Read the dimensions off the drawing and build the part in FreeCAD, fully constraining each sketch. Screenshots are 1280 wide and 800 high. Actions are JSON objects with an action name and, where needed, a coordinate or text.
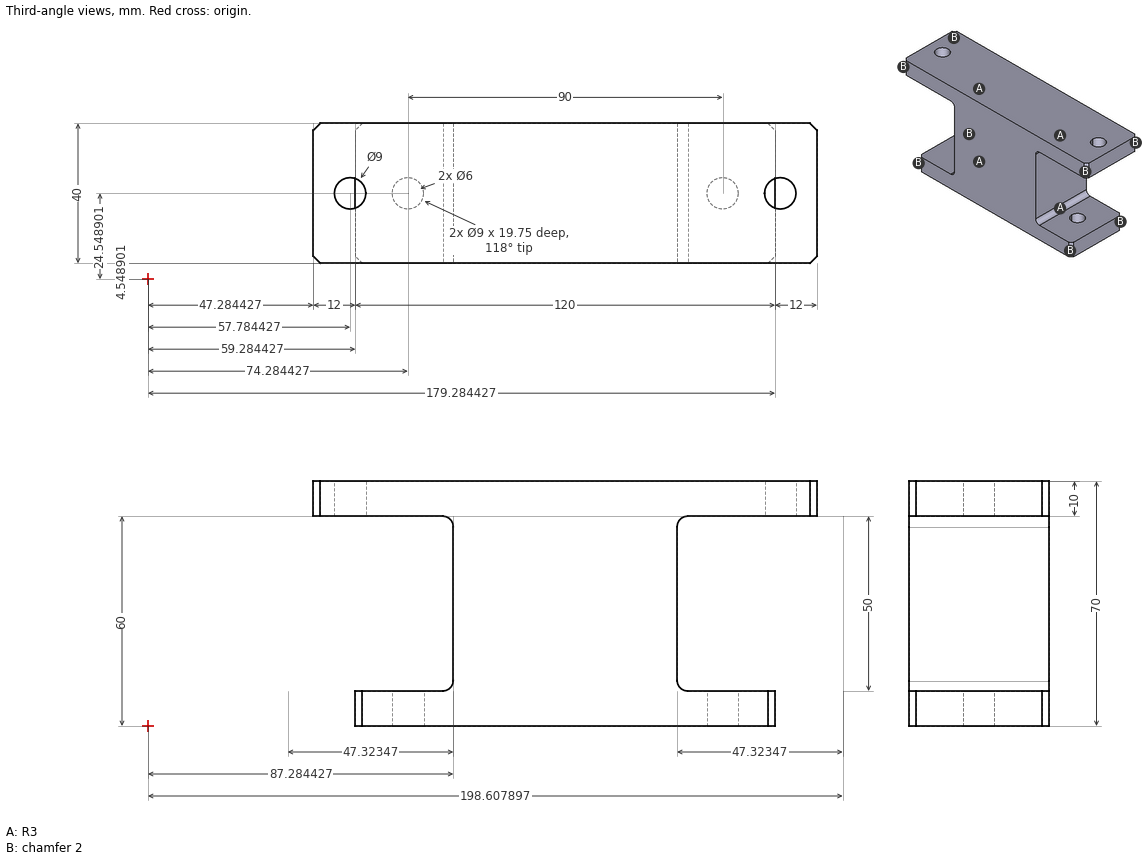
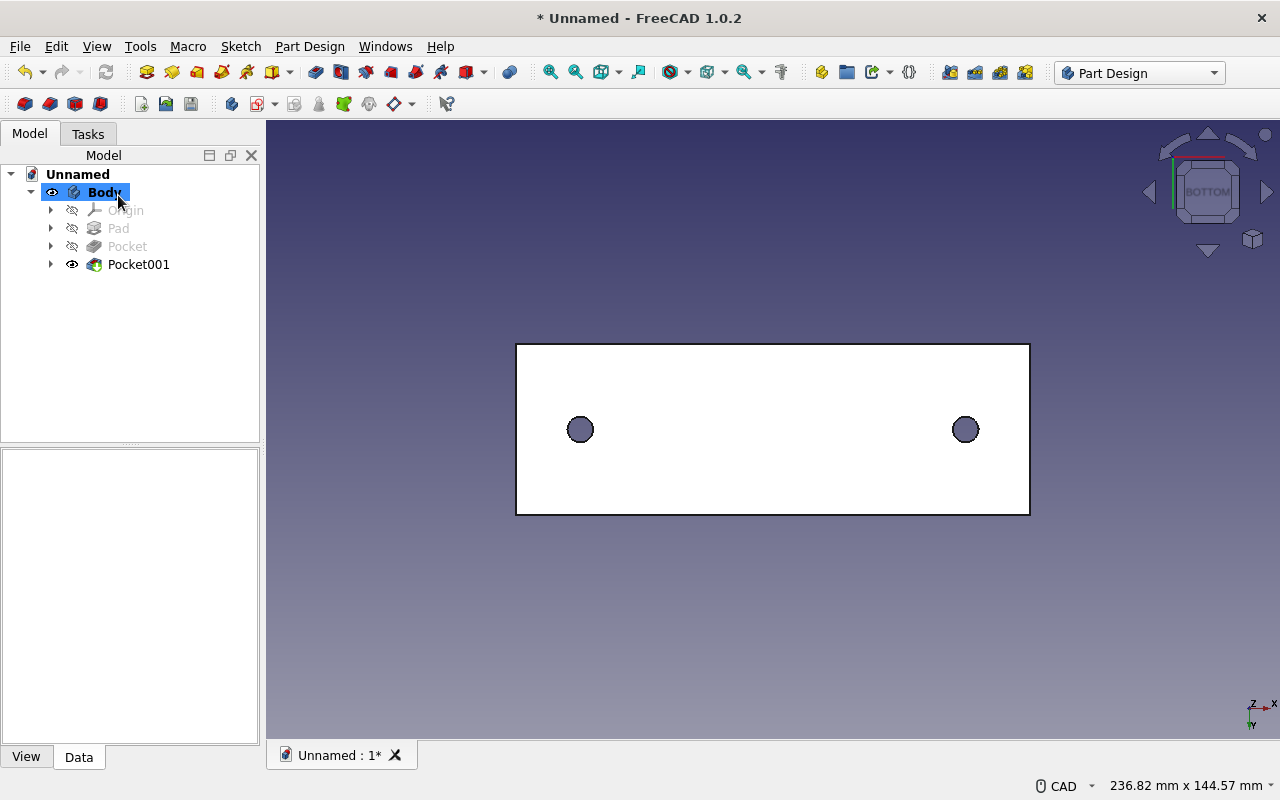
{"action": "key", "text": "4"}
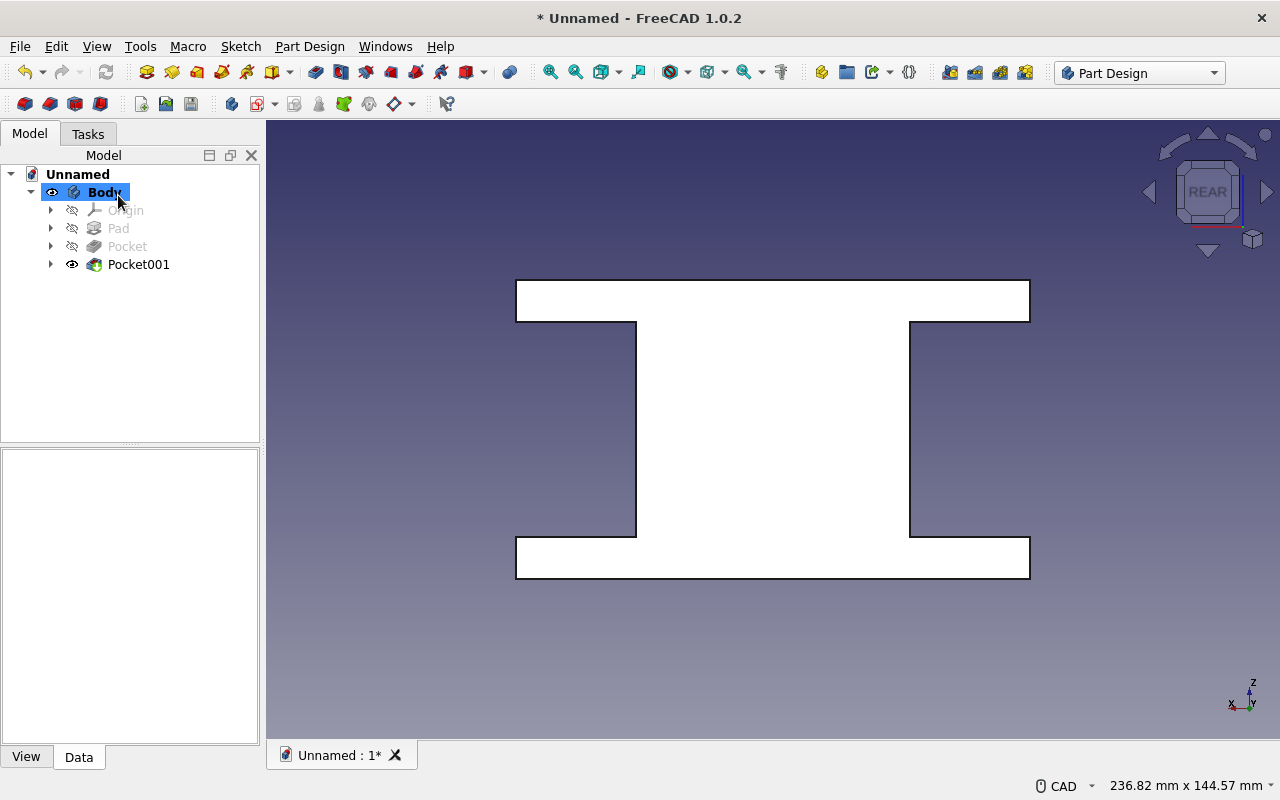
{"action": "key", "text": "6"}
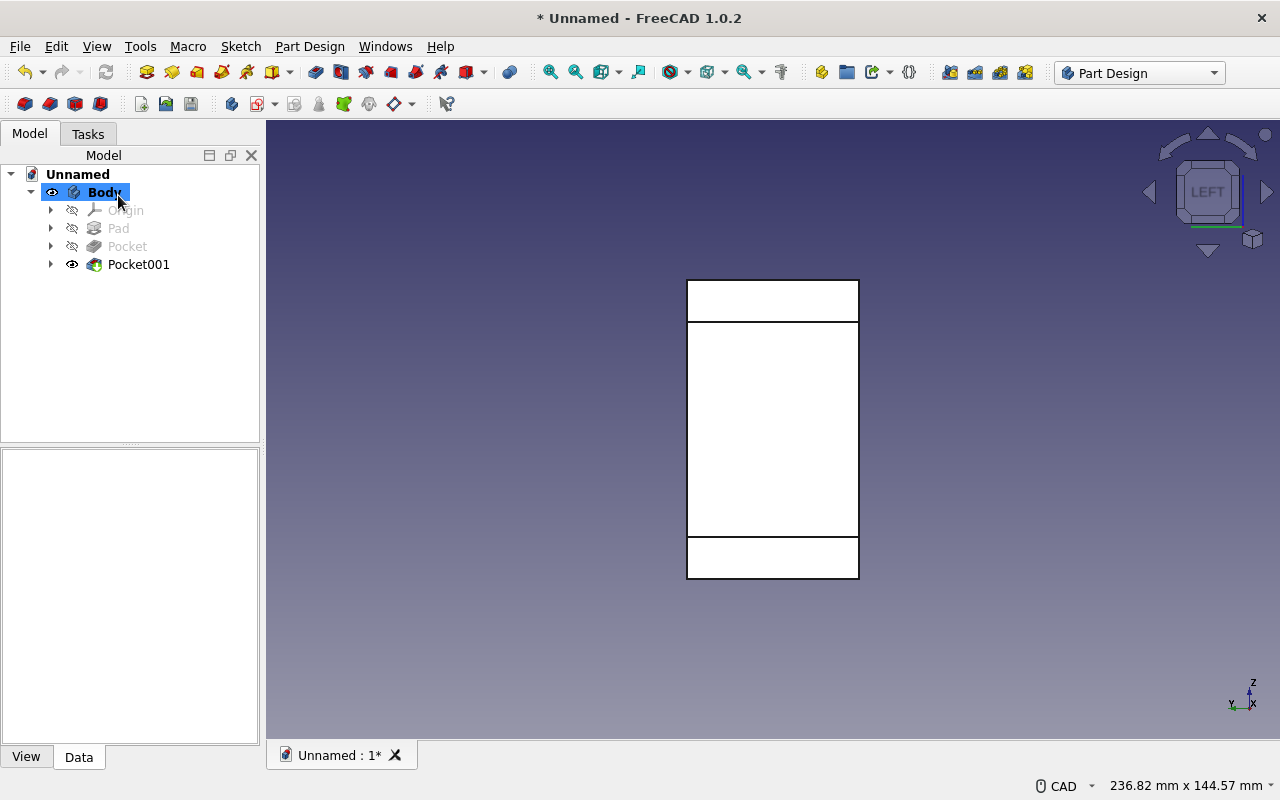
{"action": "key", "text": "v 3"}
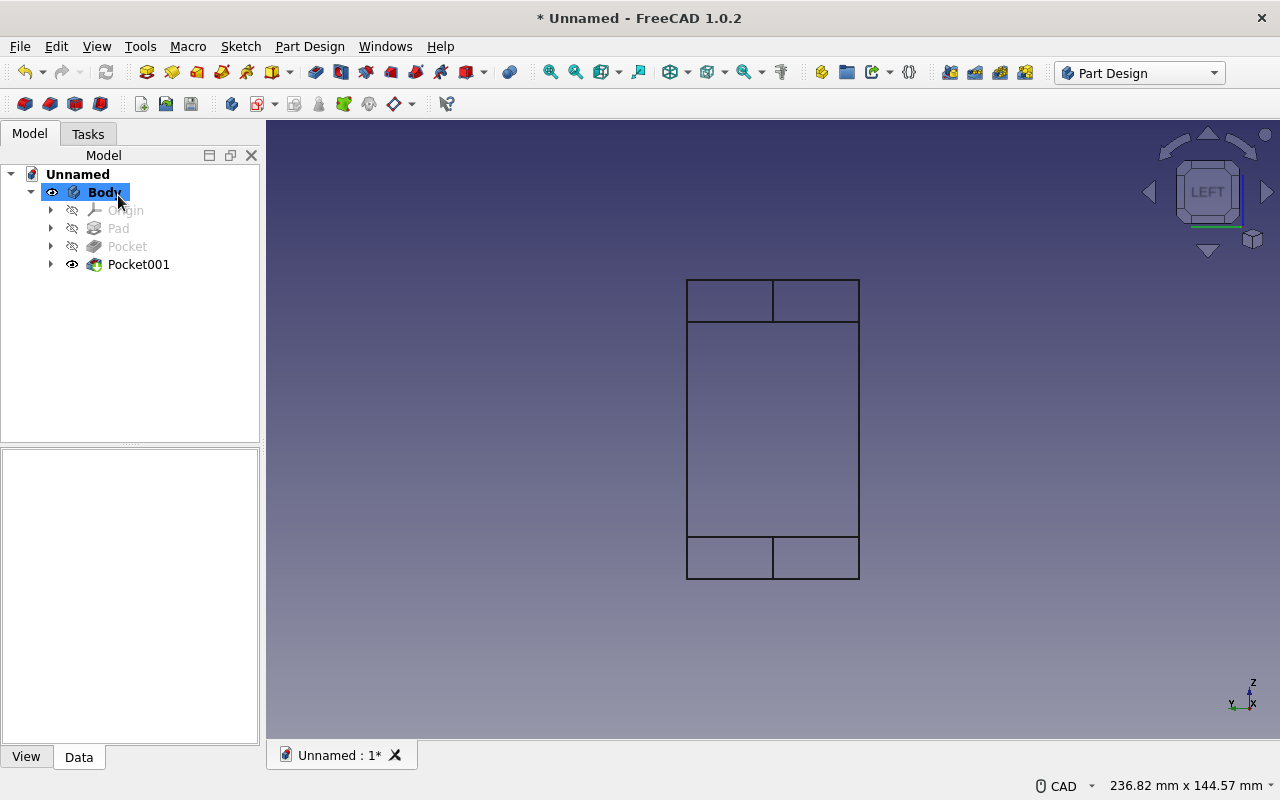
{"action": "key", "text": "0"}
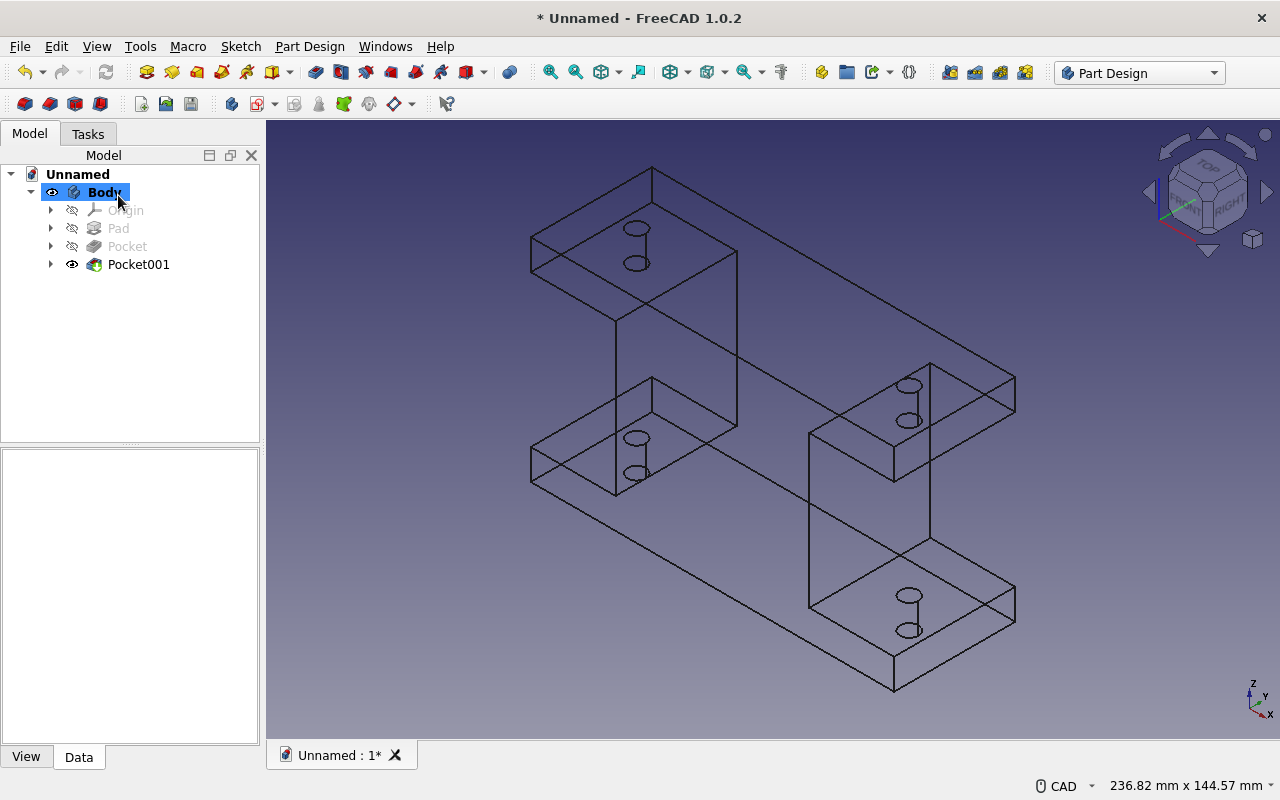
{"action": "left_click", "coordinate": [870, 572]}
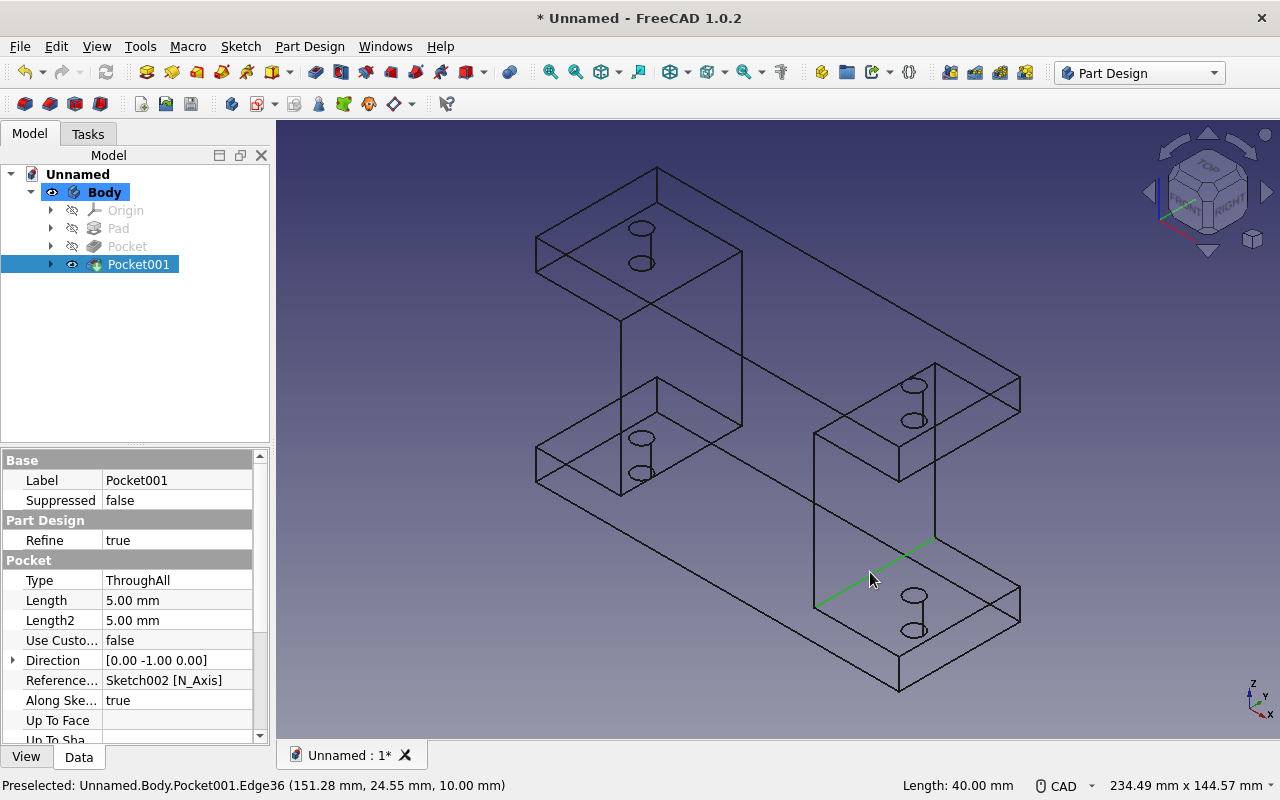
{"action": "left_click", "coordinate": [875, 397], "text": "ctrl"}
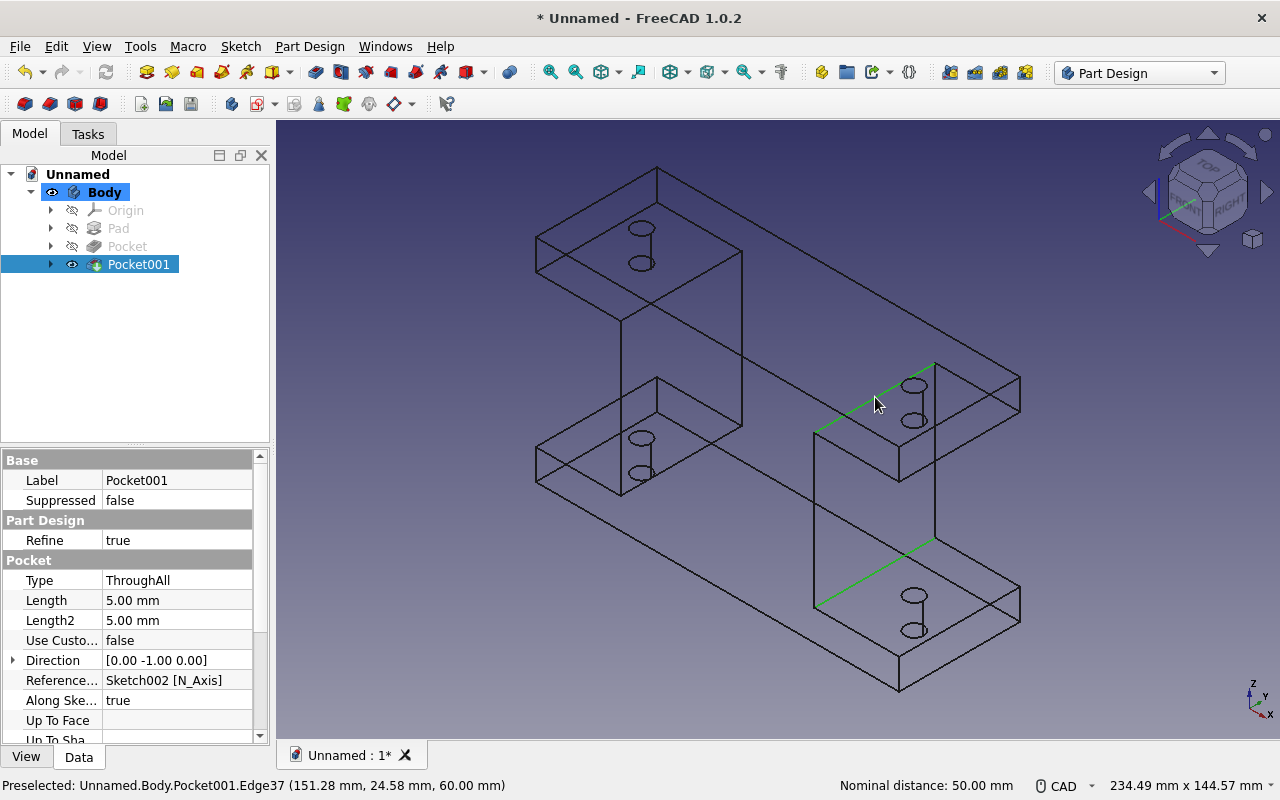
{"action": "left_click", "coordinate": [681, 285], "text": "ctrl"}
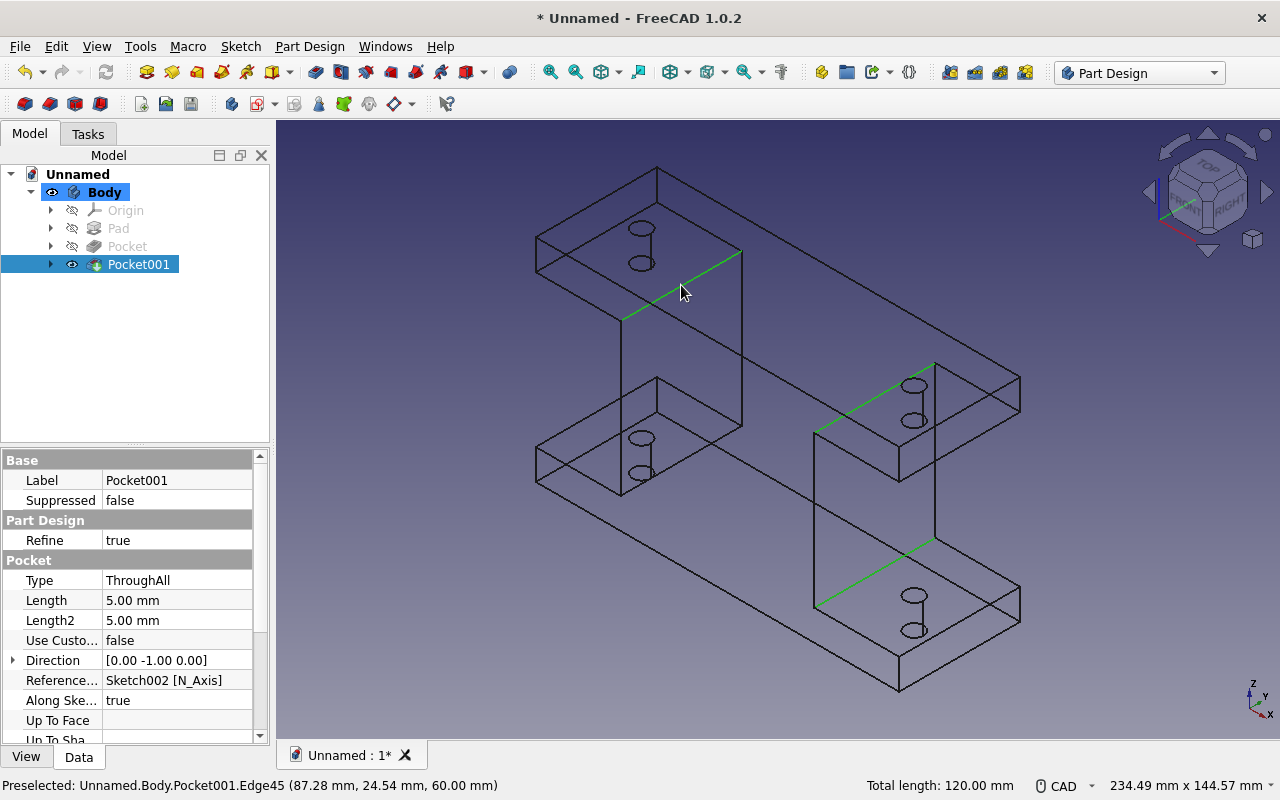
{"action": "left_click", "coordinate": [681, 460], "text": "ctrl"}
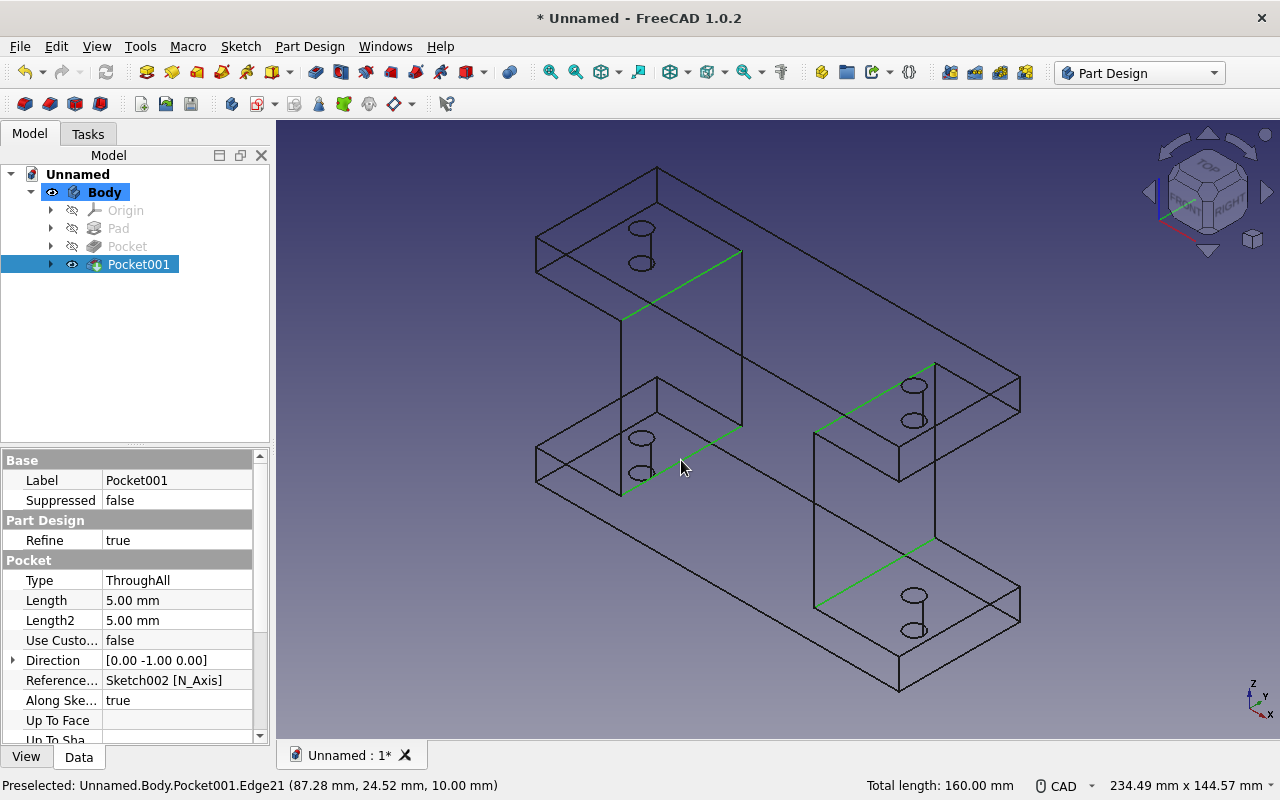
{"action": "key", "text": "v 1"}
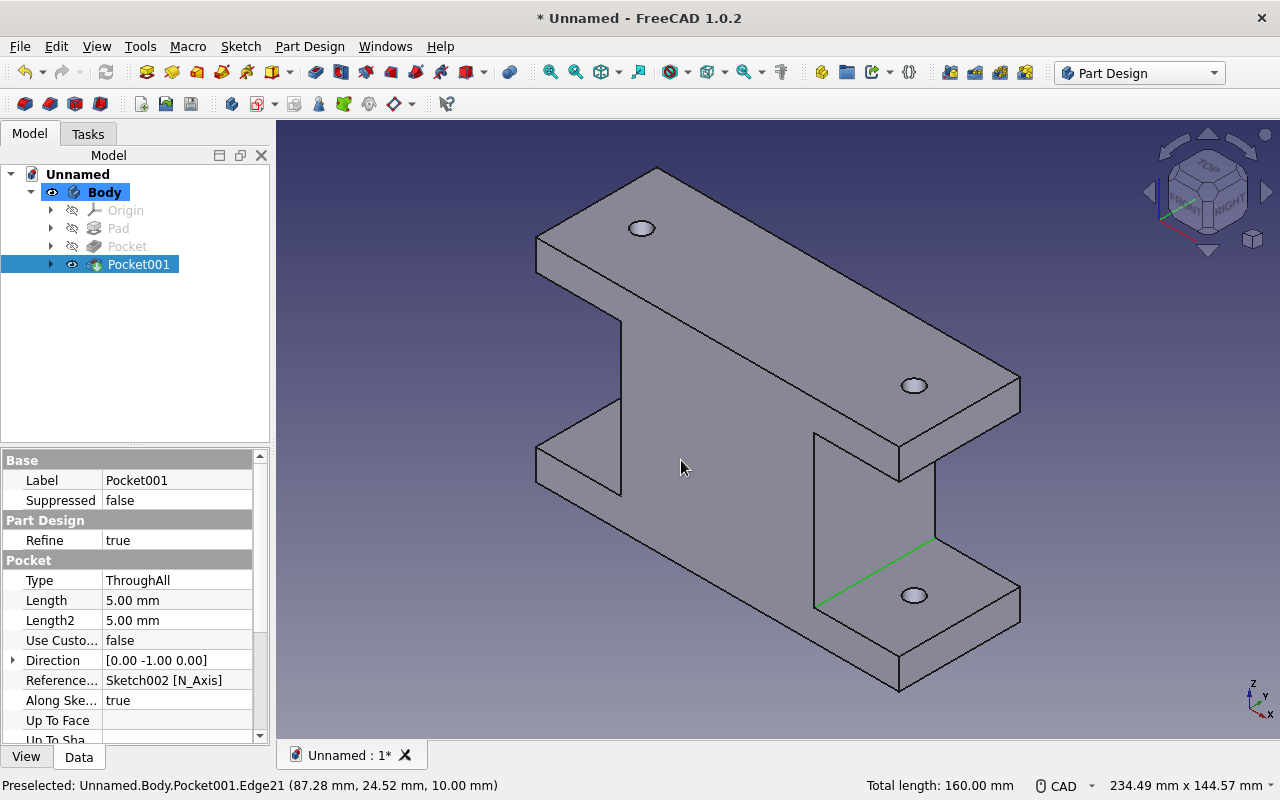
{"action": "left_click", "coordinate": [25, 104]}